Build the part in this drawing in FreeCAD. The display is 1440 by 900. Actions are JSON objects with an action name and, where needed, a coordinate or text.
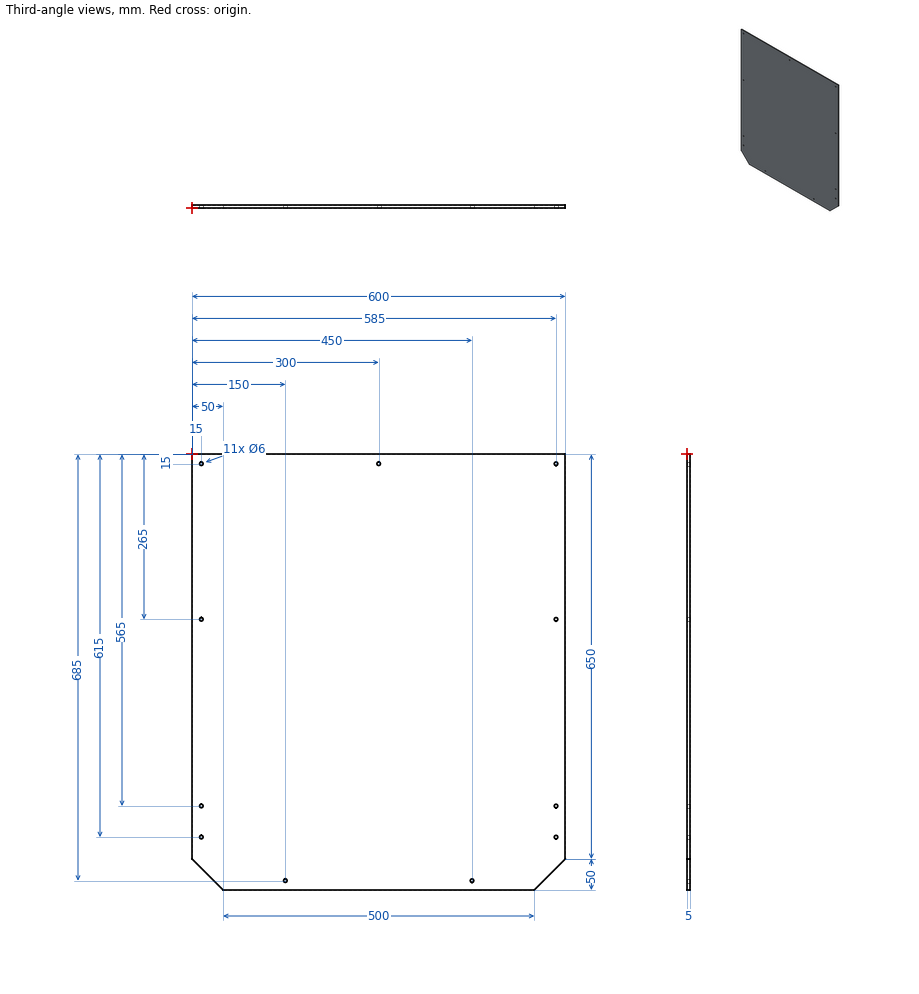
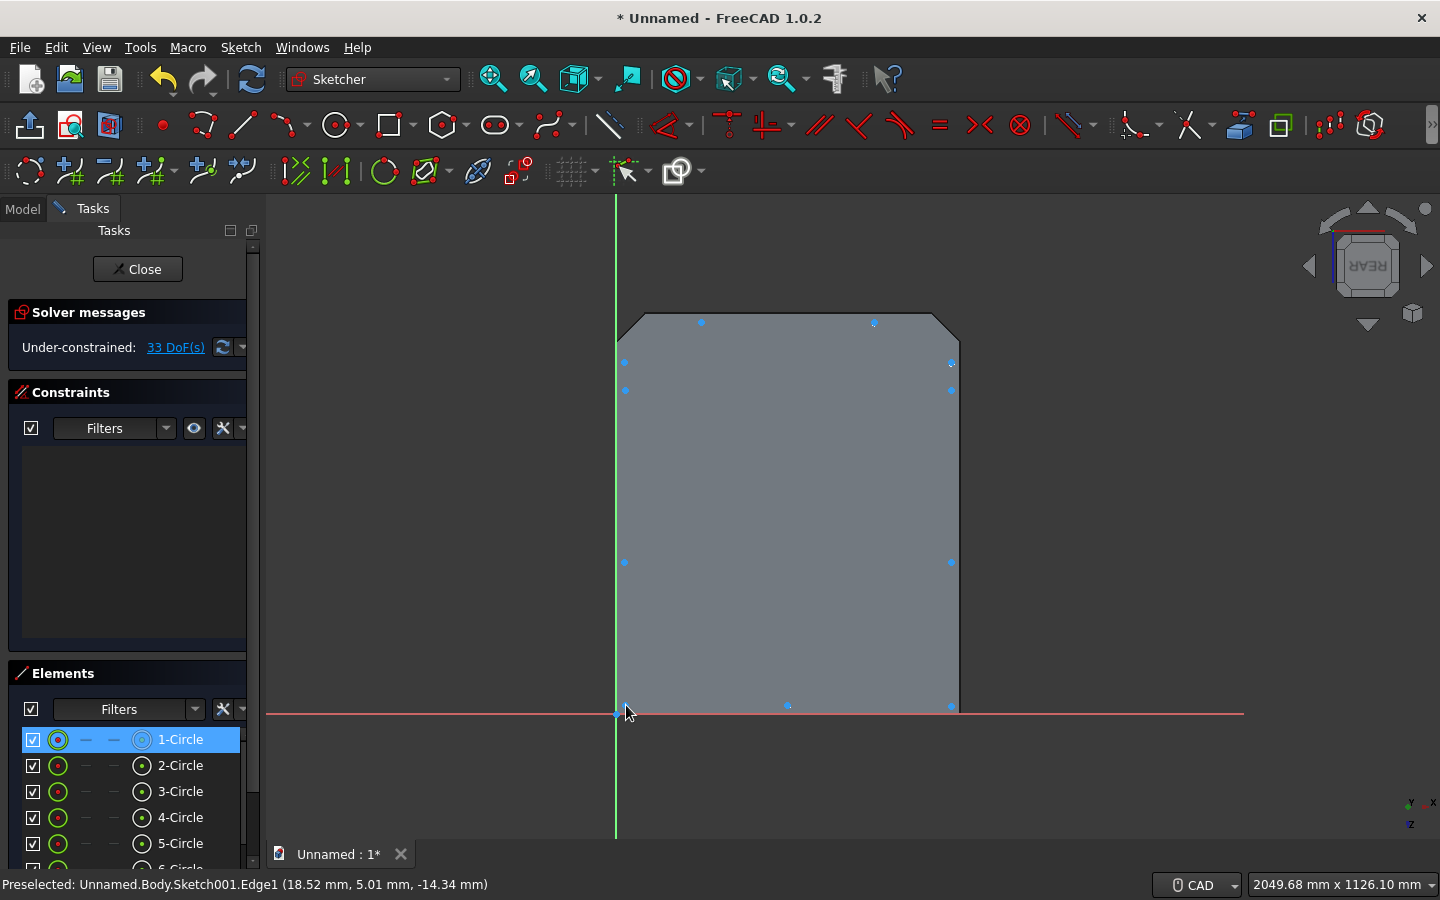
{"action": "scroll", "coordinate": [626, 561], "scroll_direction": "up", "scroll_amount": 10}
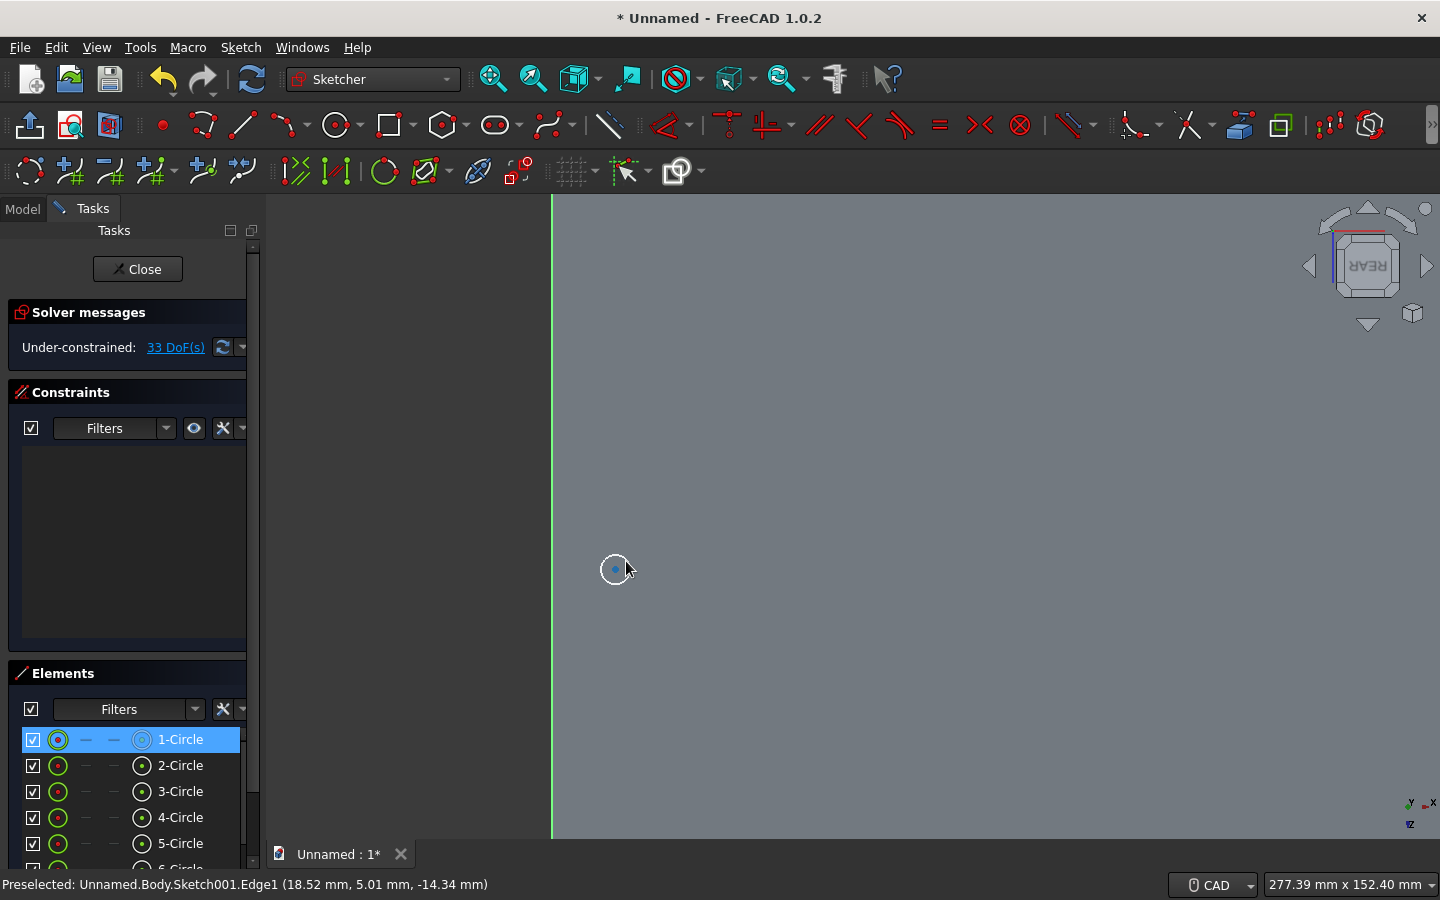
{"action": "left_click", "coordinate": [626, 559]}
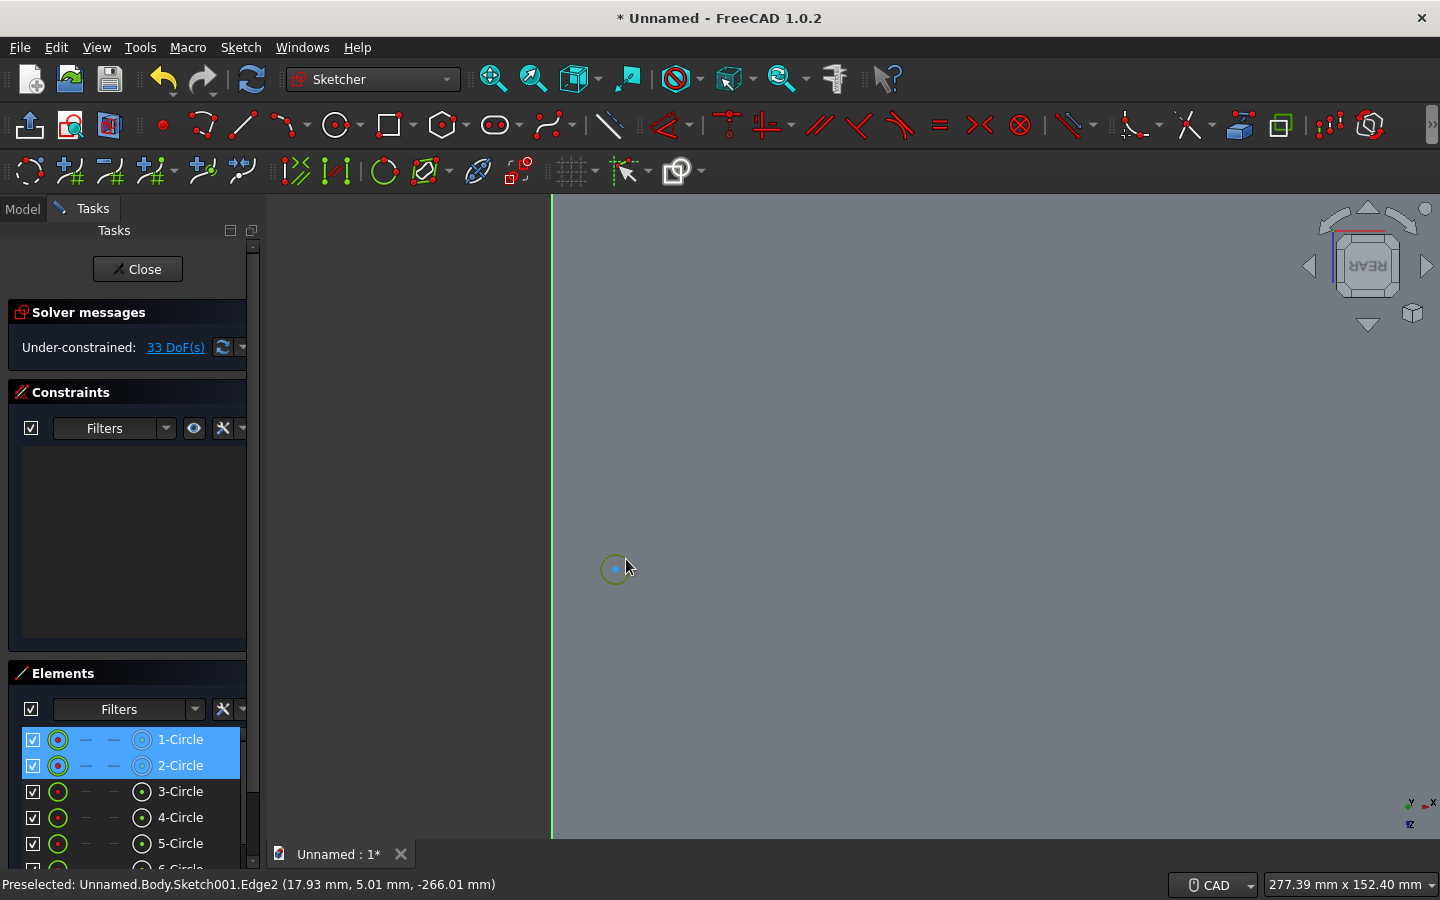
{"action": "scroll", "coordinate": [626, 561], "scroll_direction": "down", "scroll_amount": 10}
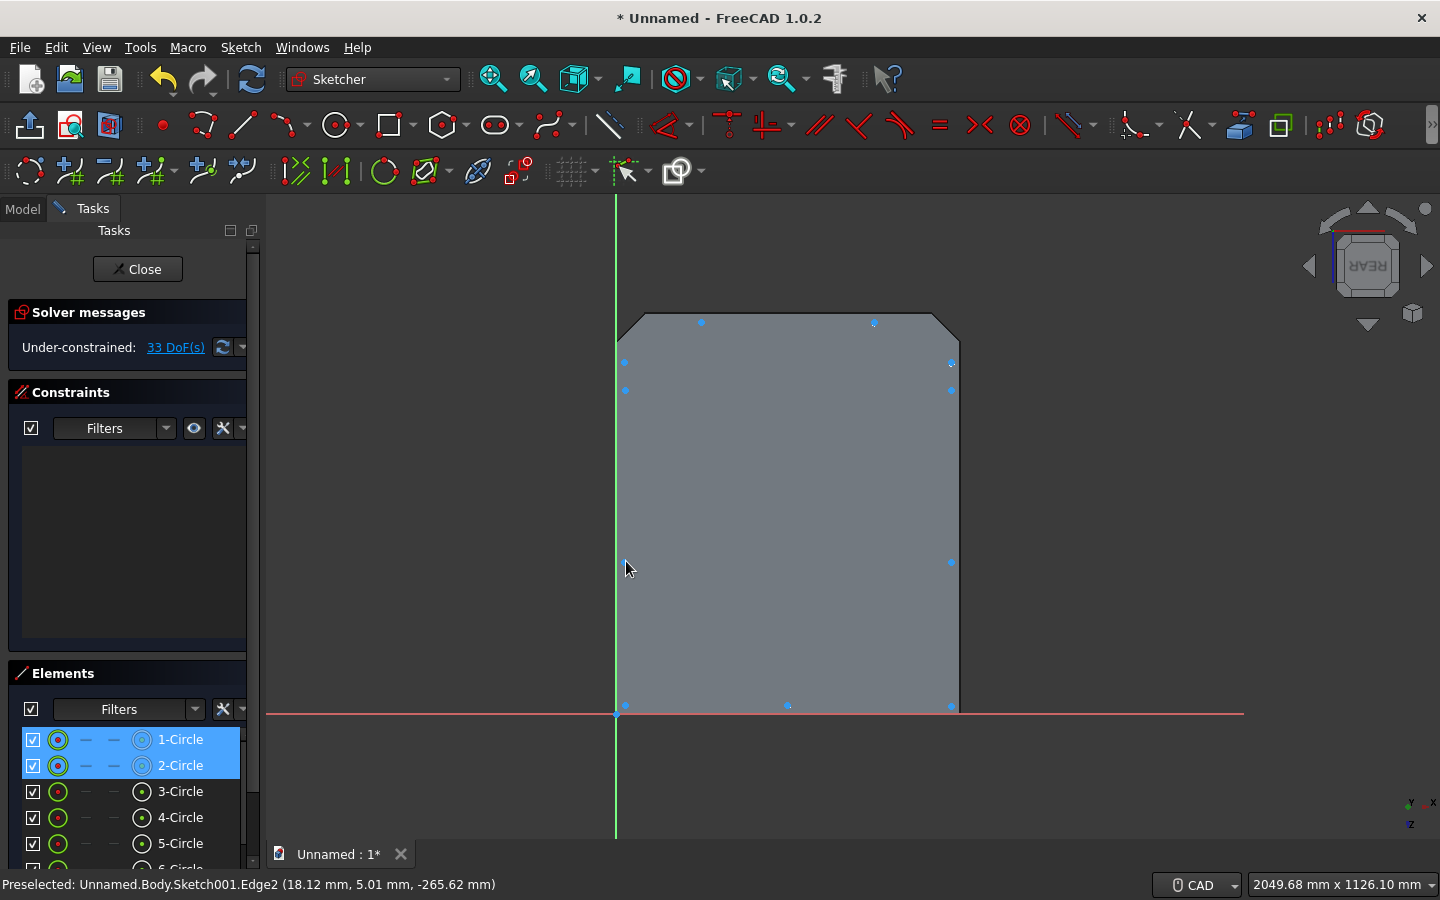
{"action": "scroll", "coordinate": [626, 390], "scroll_direction": "up", "scroll_amount": 11}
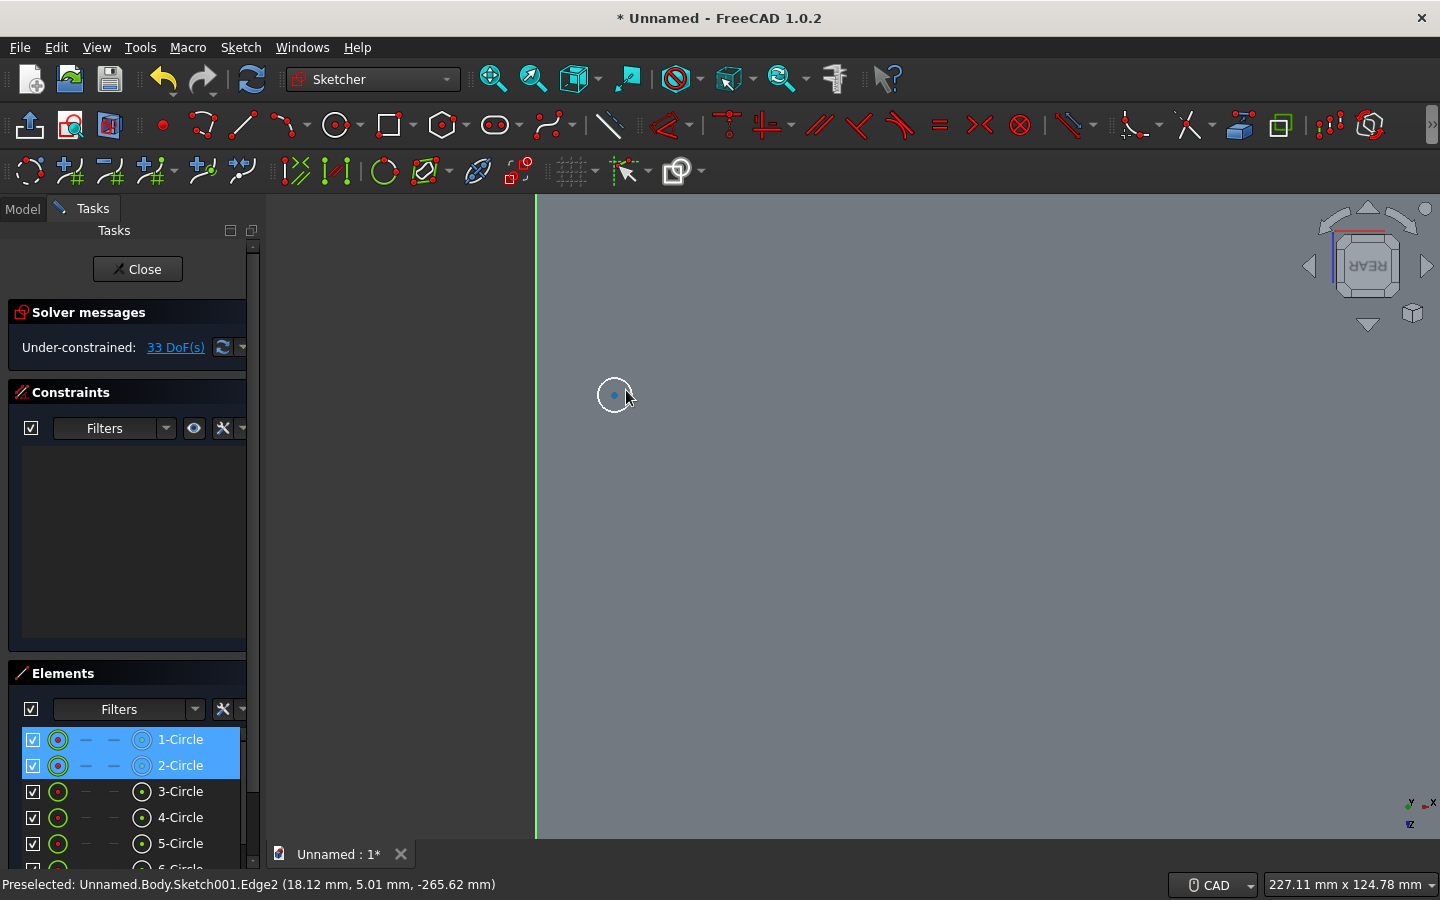
{"action": "left_click", "coordinate": [627, 383]}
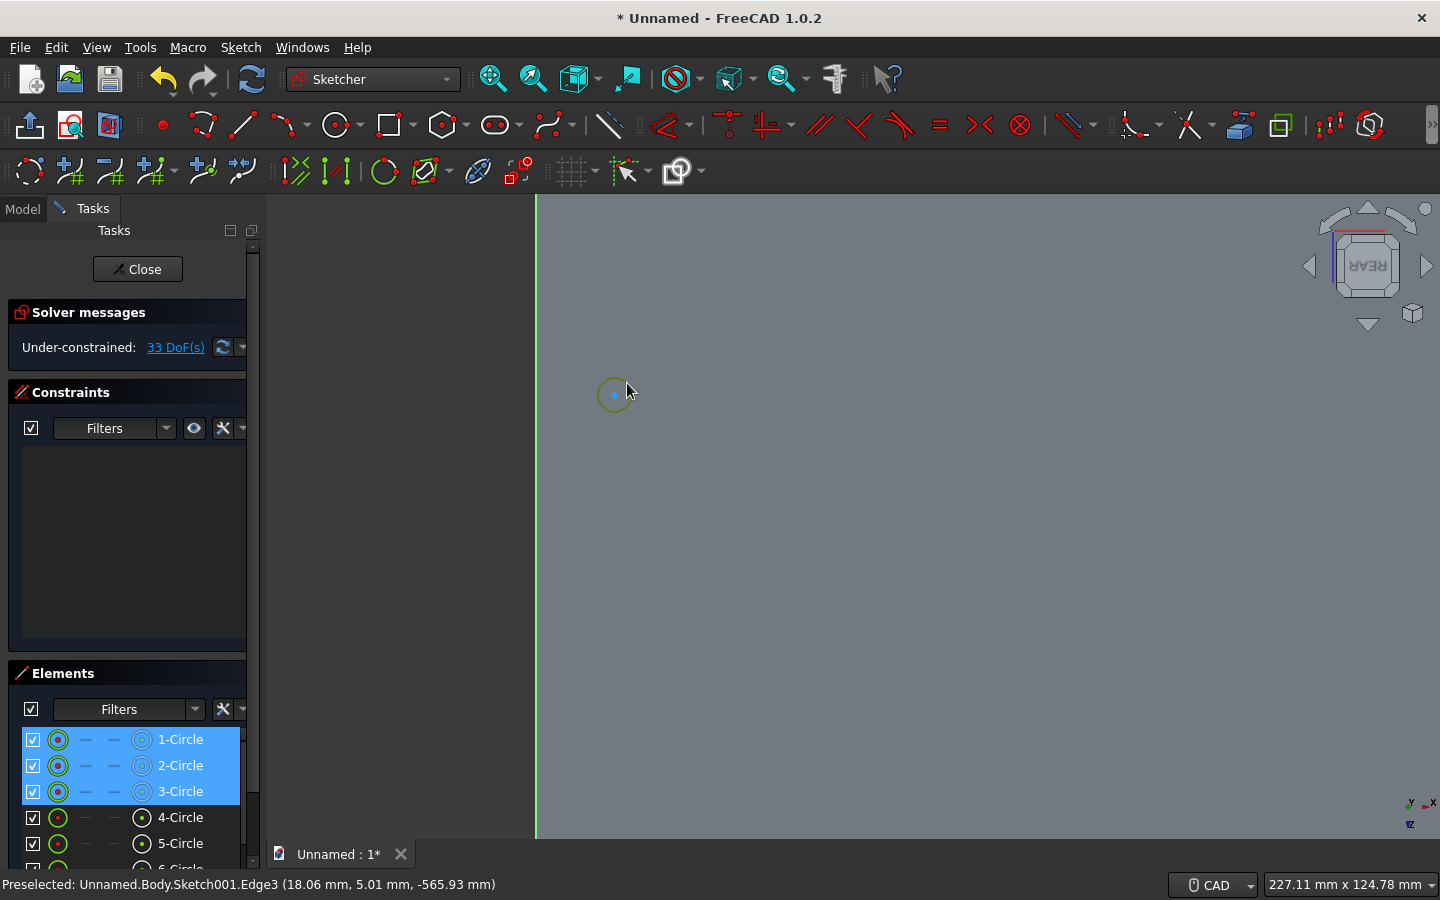
{"action": "scroll", "coordinate": [626, 390], "scroll_direction": "down", "scroll_amount": 11}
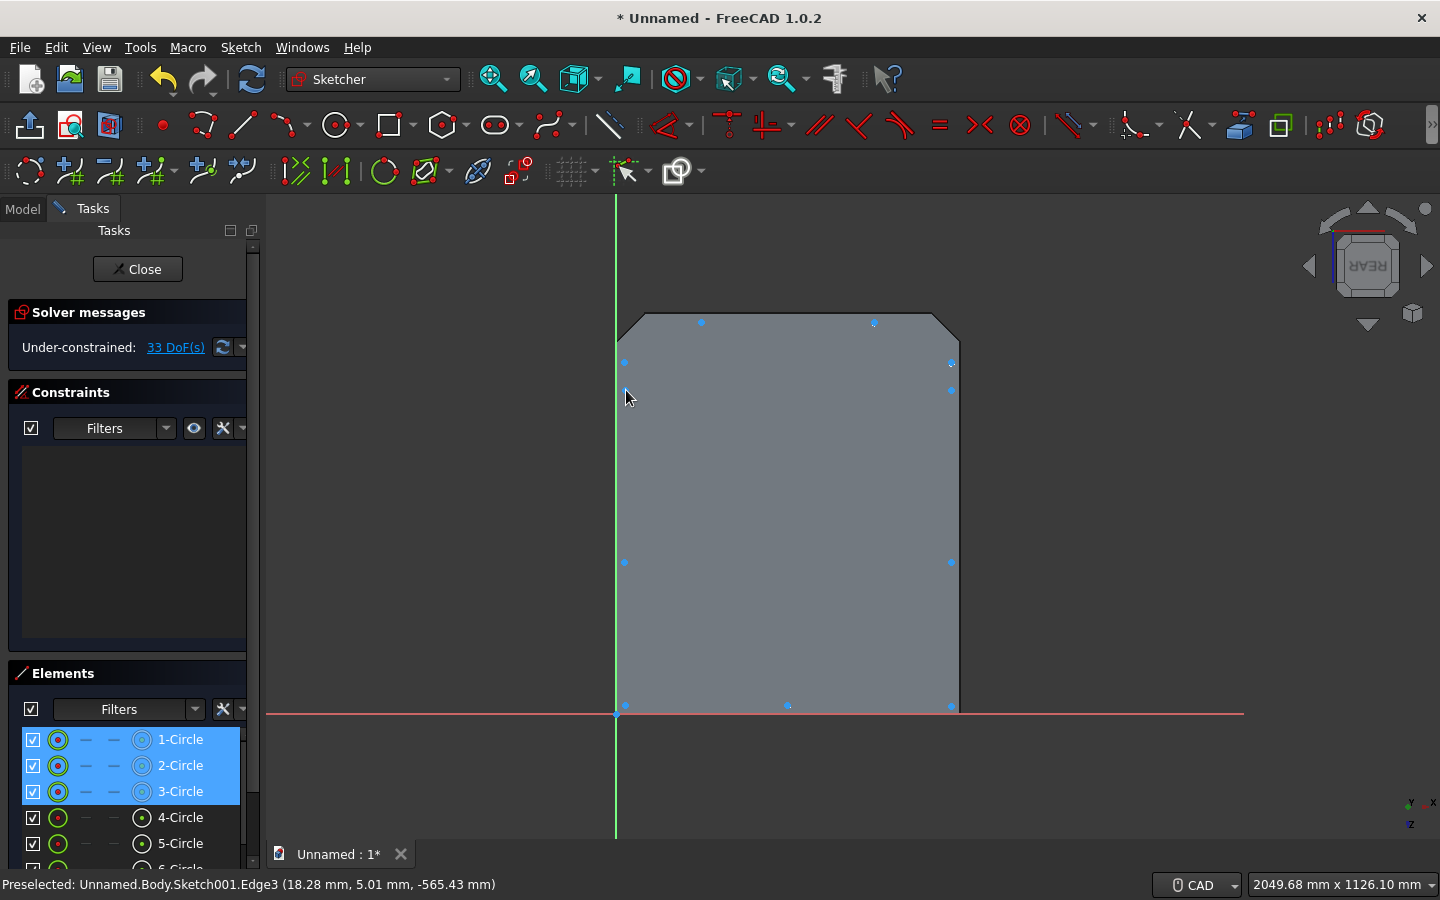
{"action": "scroll", "coordinate": [626, 361], "scroll_direction": "up", "scroll_amount": 10}